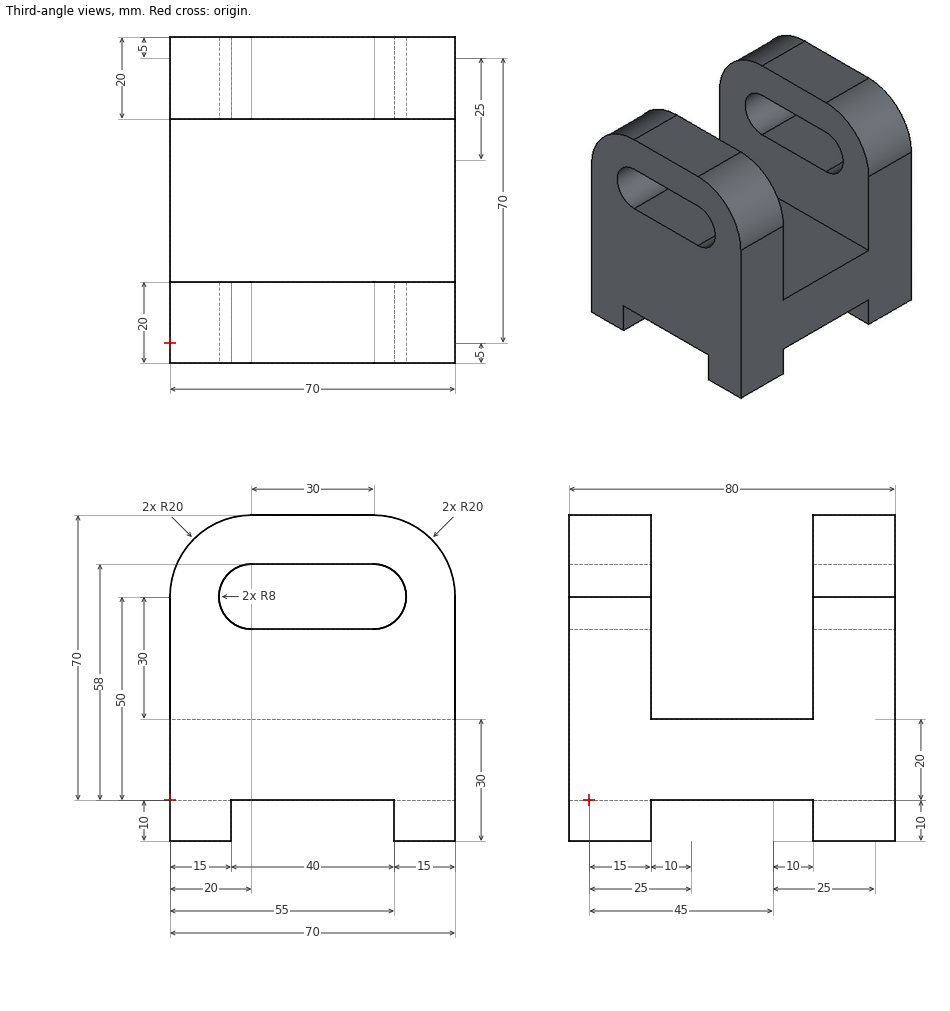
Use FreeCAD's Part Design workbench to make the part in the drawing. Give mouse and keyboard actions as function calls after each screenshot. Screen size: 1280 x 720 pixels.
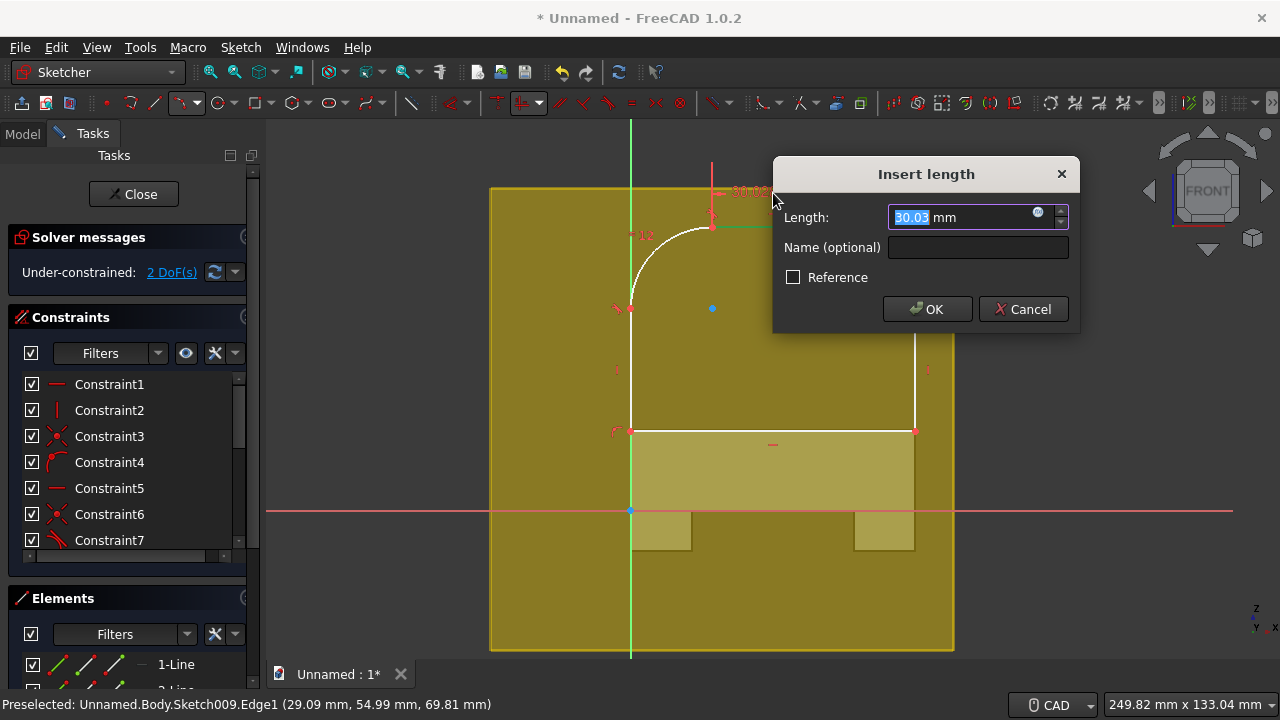
text(30)
key(Return)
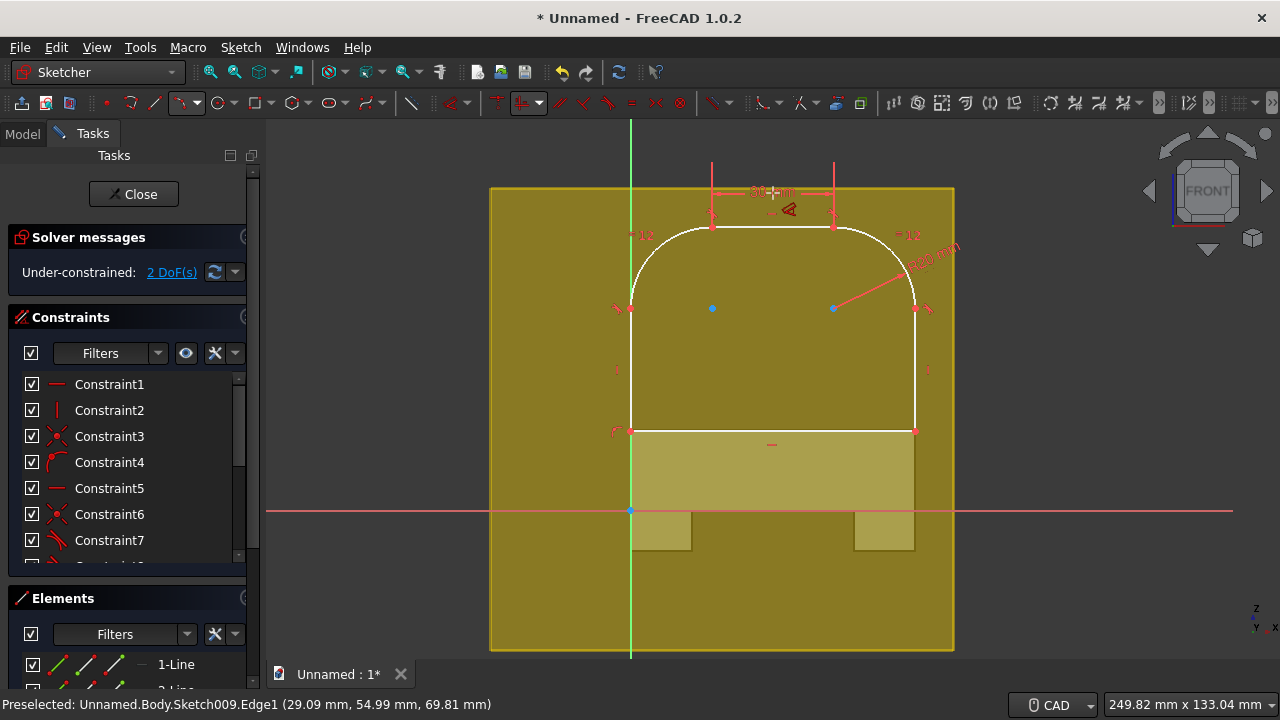
click(915, 345)
click(949, 370)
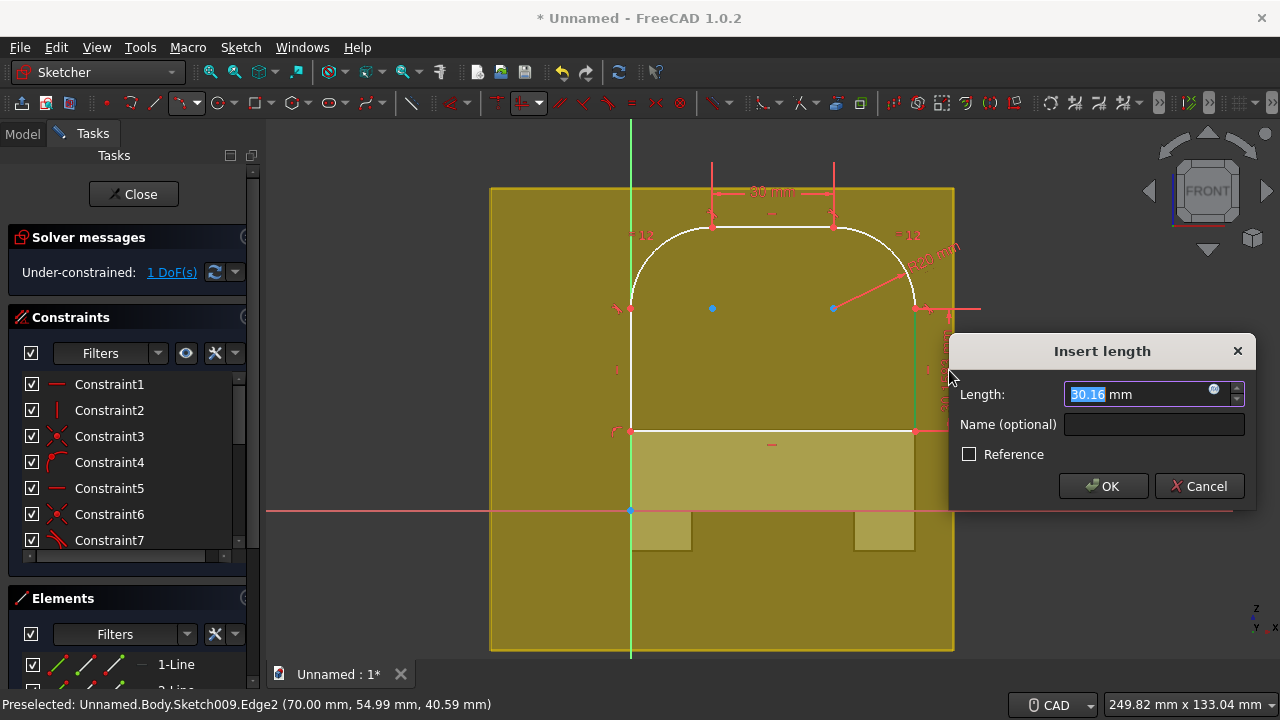
text(30)
key(Return)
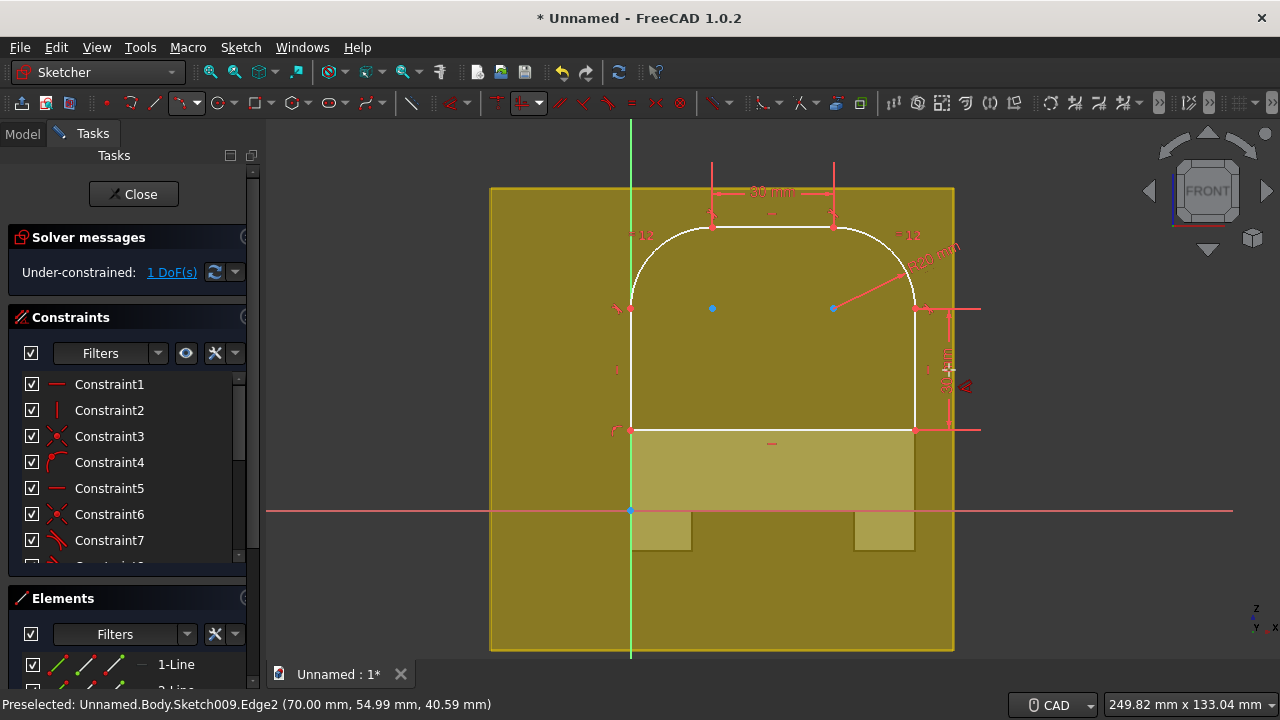
click(712, 227)
click(597, 369)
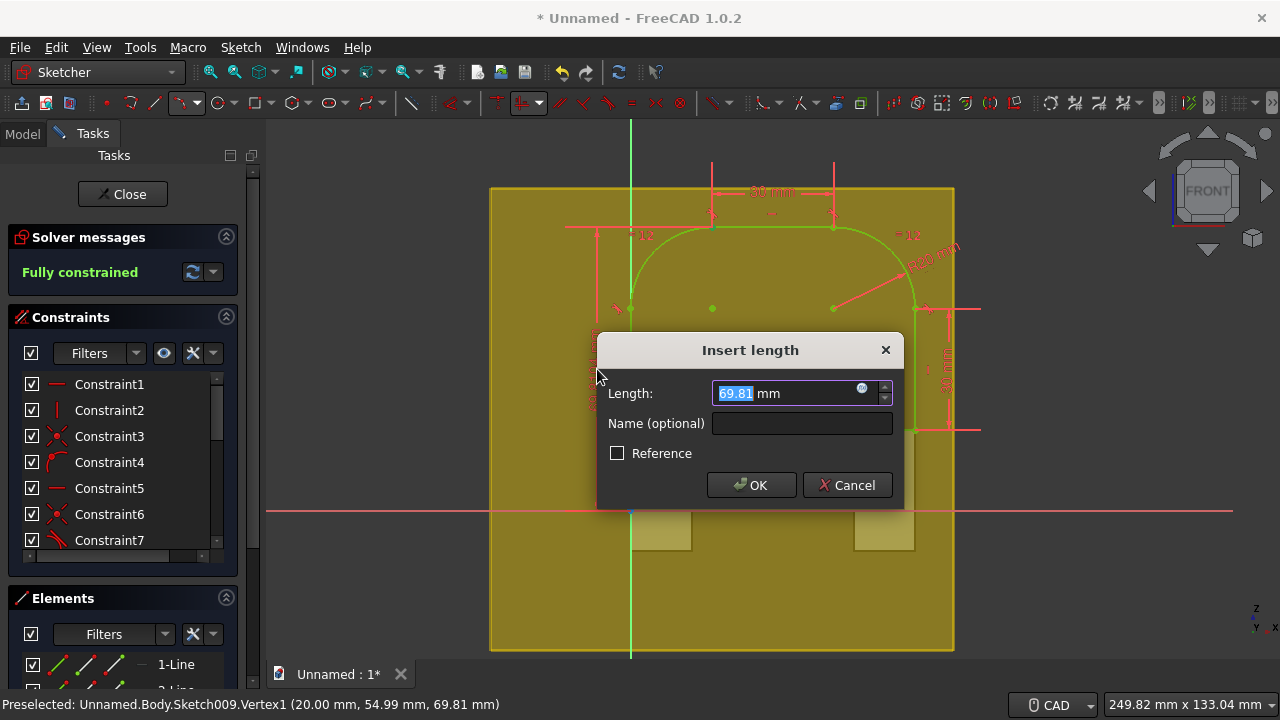
text(70)
key(Return)
key(Escape)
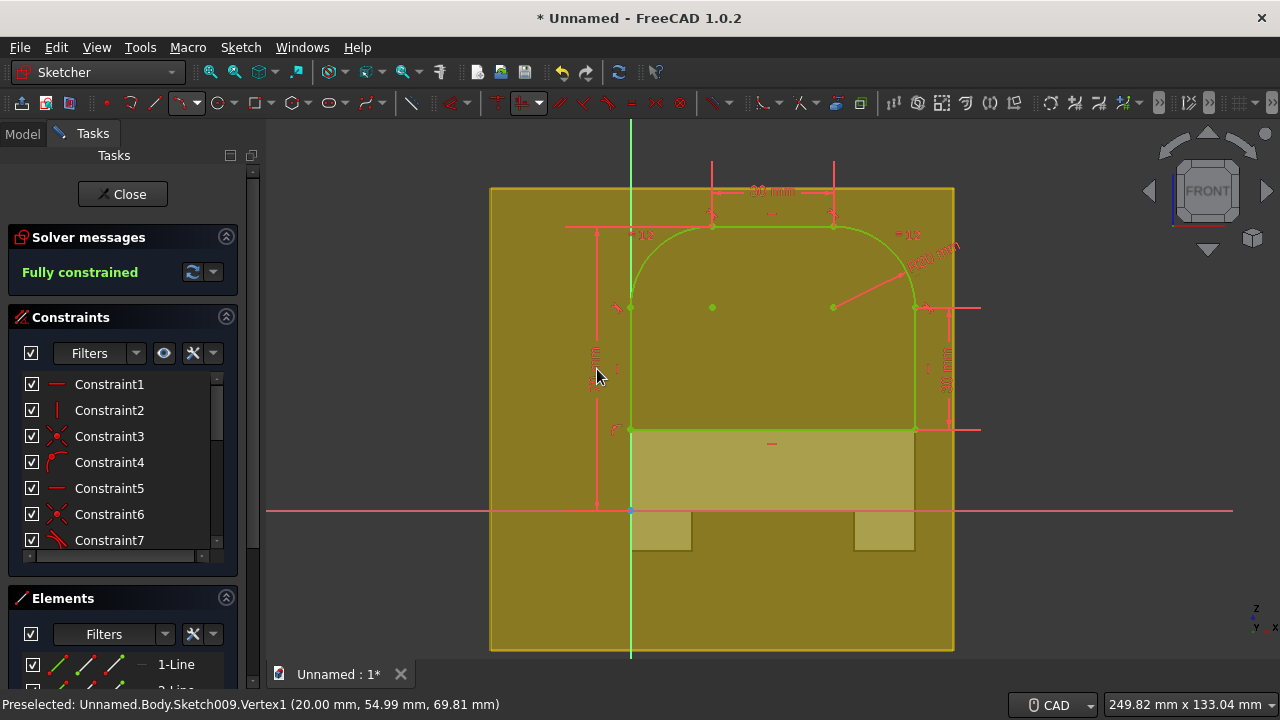
click(123, 194)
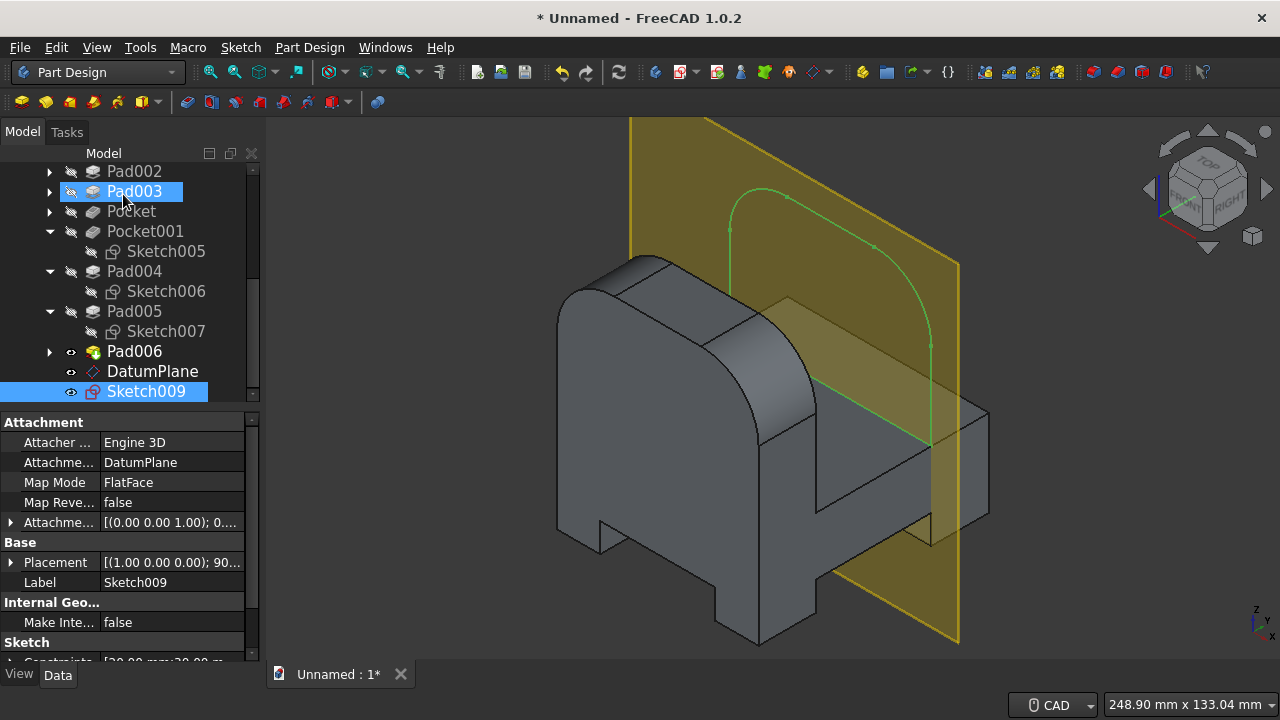
click(22, 102)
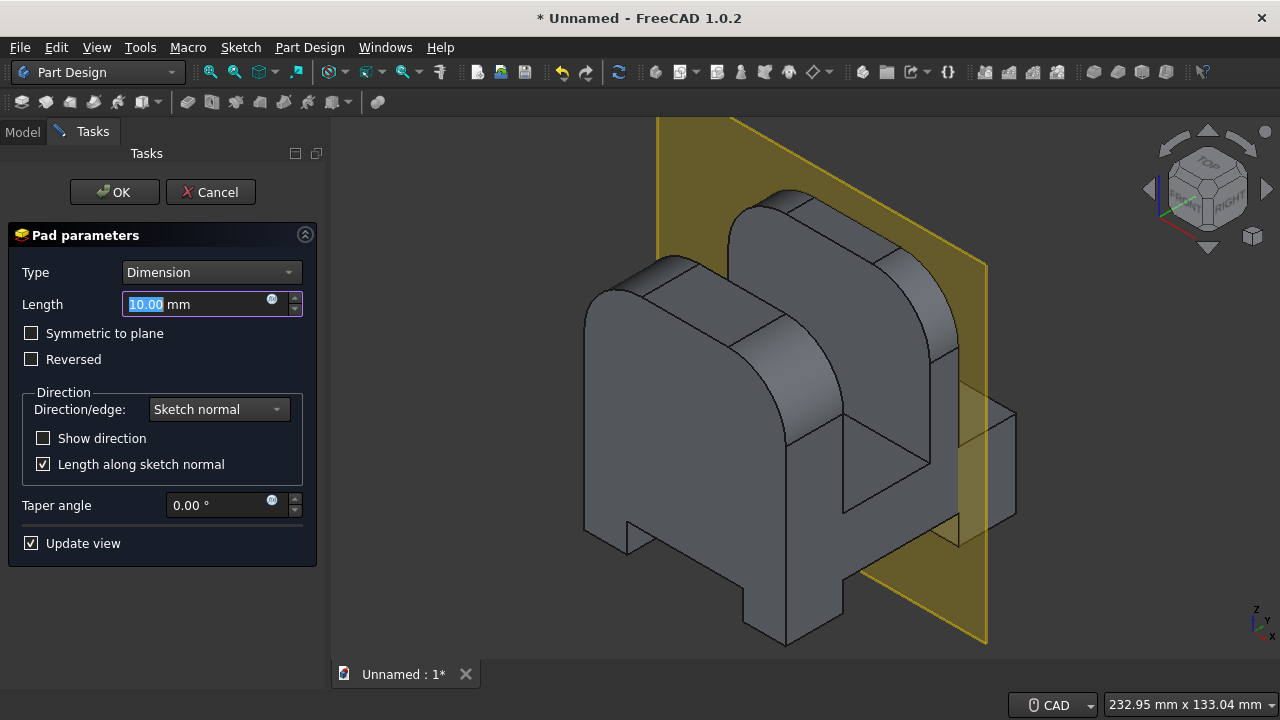
text(20)
key(Tab)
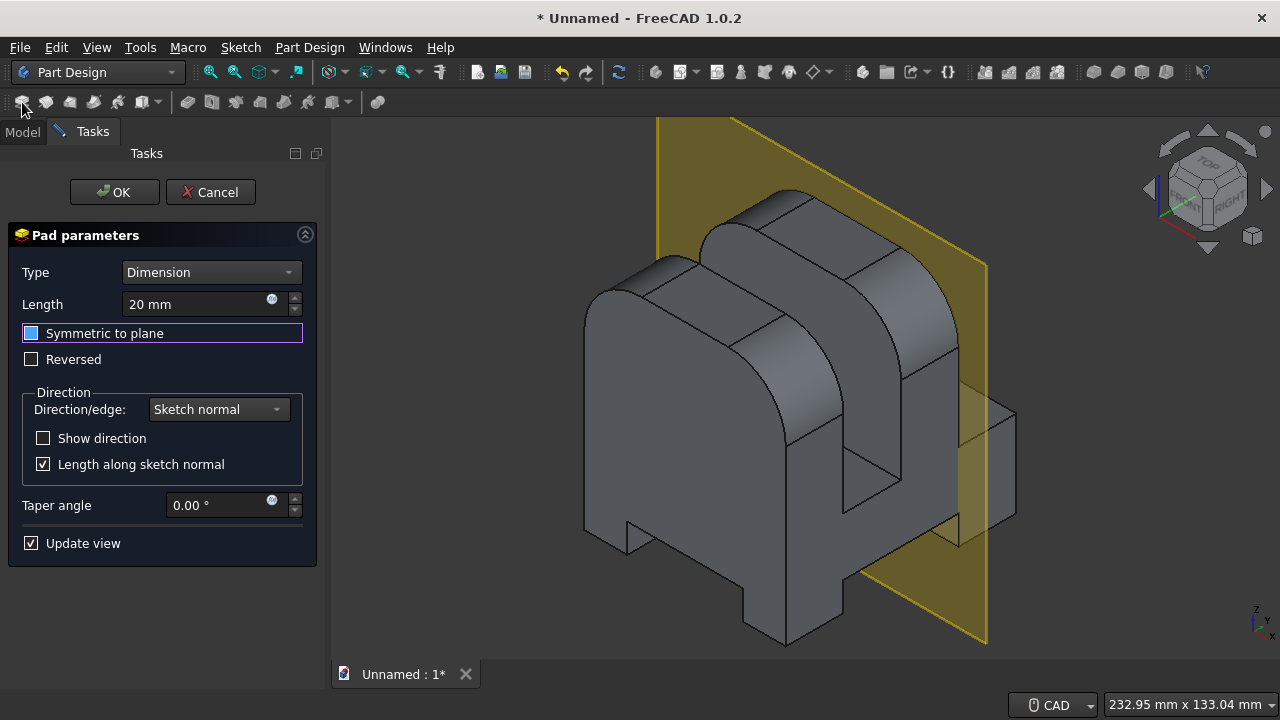
click(30, 359)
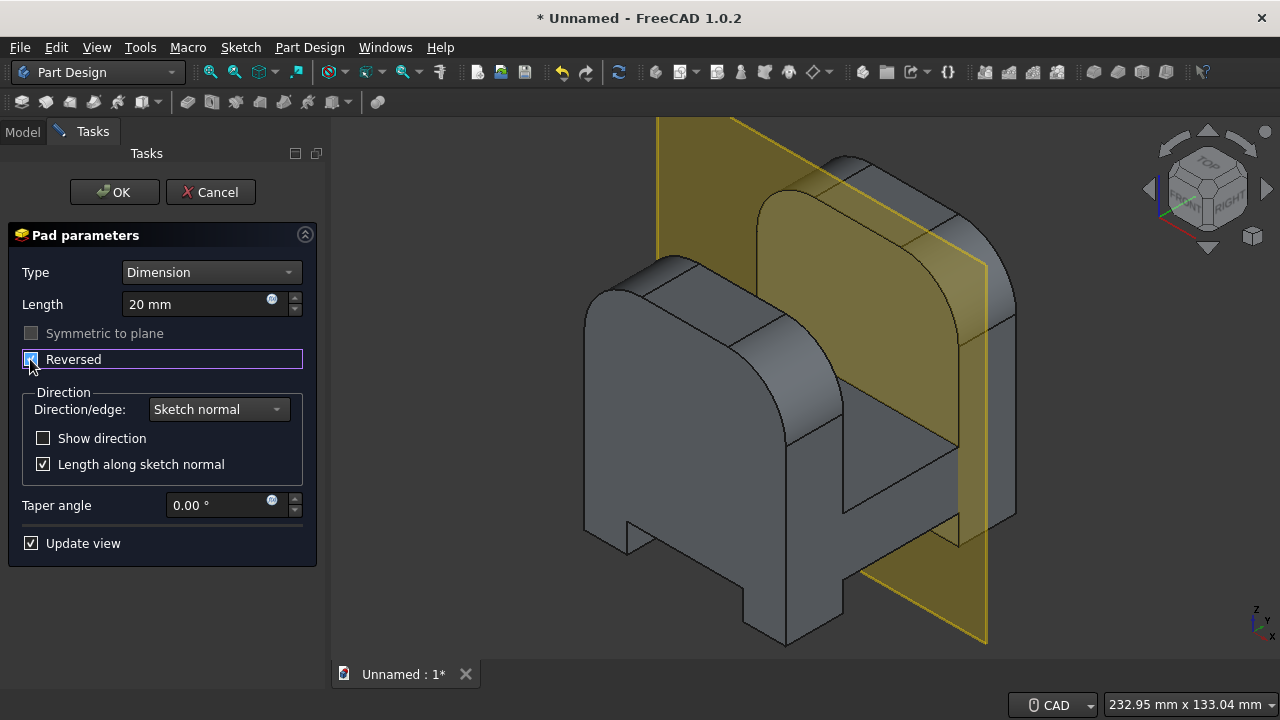
click(115, 192)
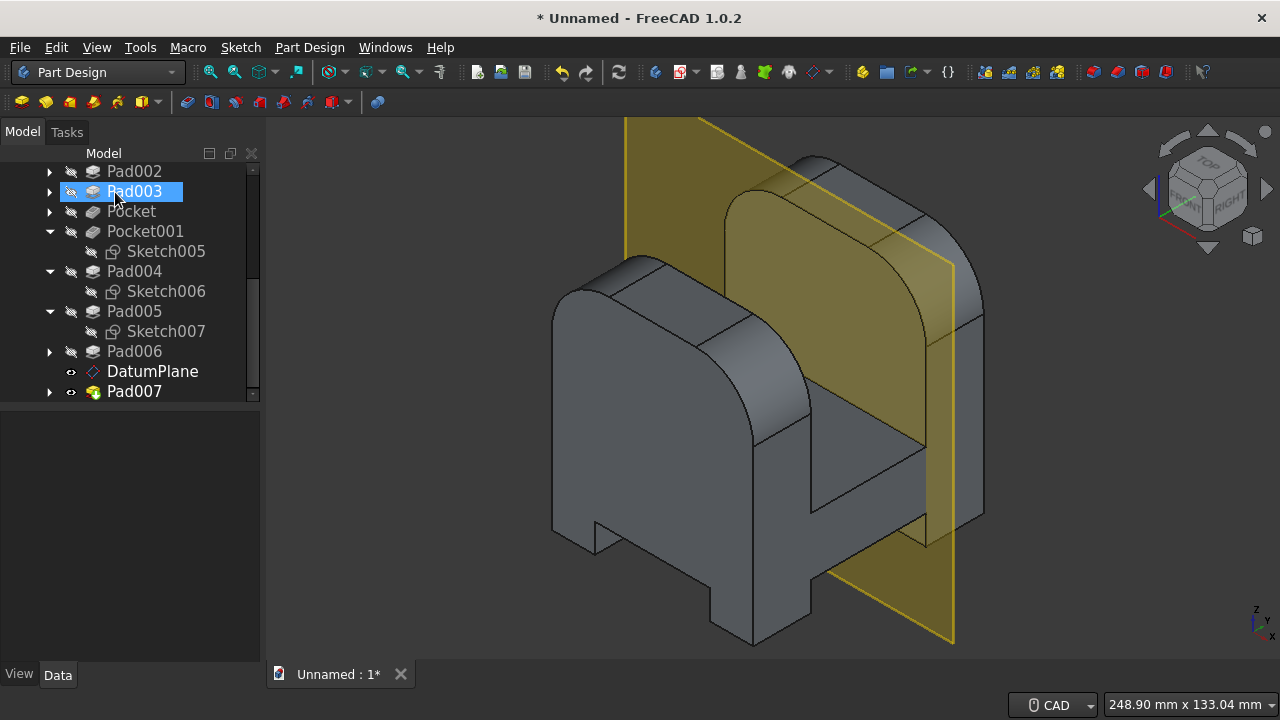
click(116, 372)
key(space)